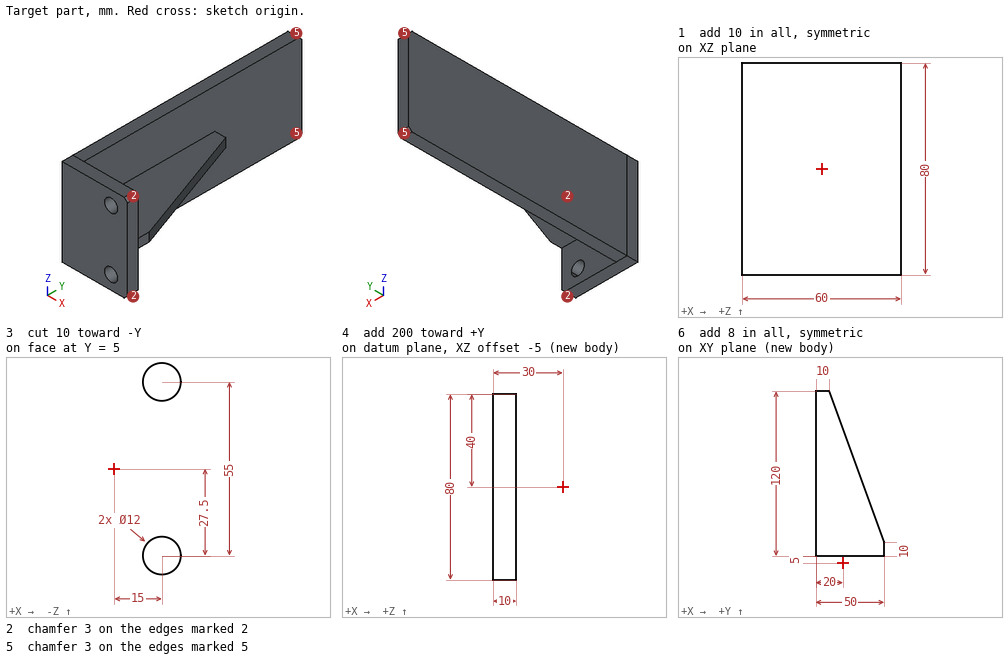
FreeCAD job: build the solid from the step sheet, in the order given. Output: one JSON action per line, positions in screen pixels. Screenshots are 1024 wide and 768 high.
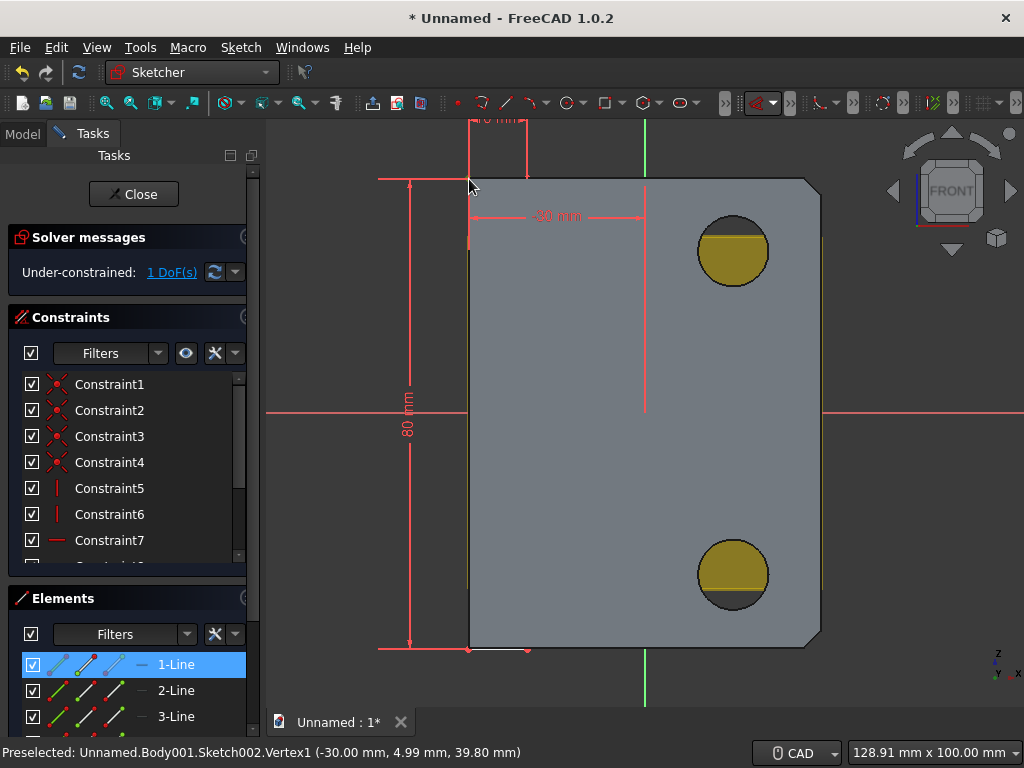
{"action": "key", "text": "i"}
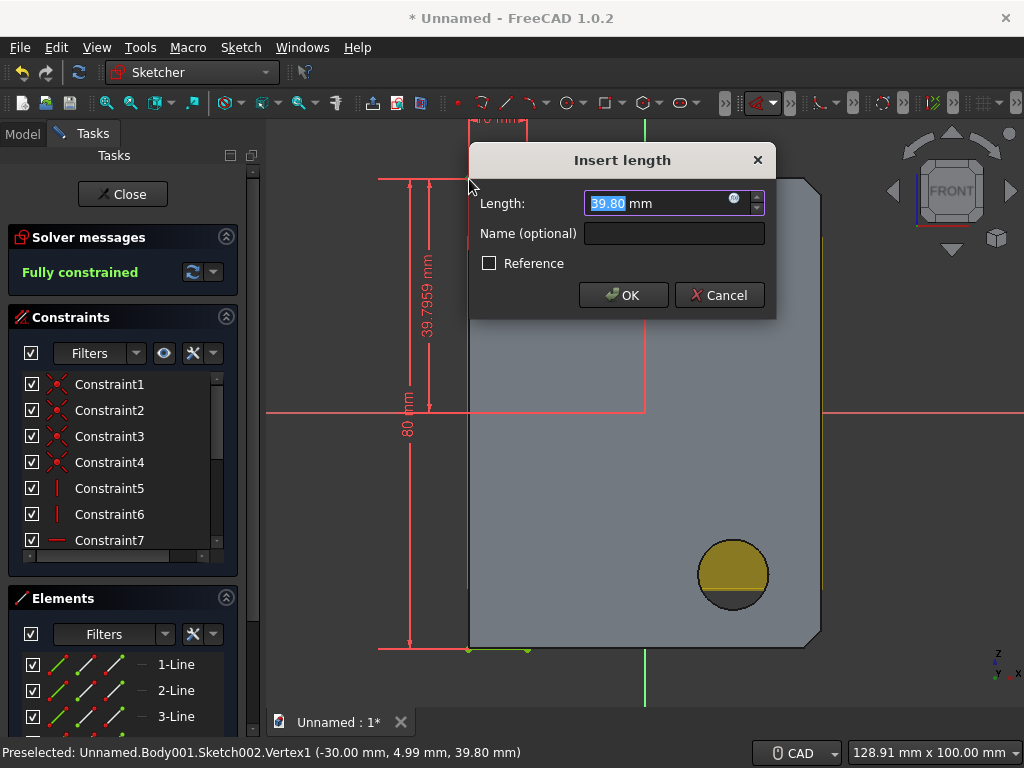
{"action": "type", "text": "40"}
{"action": "key", "text": "Return"}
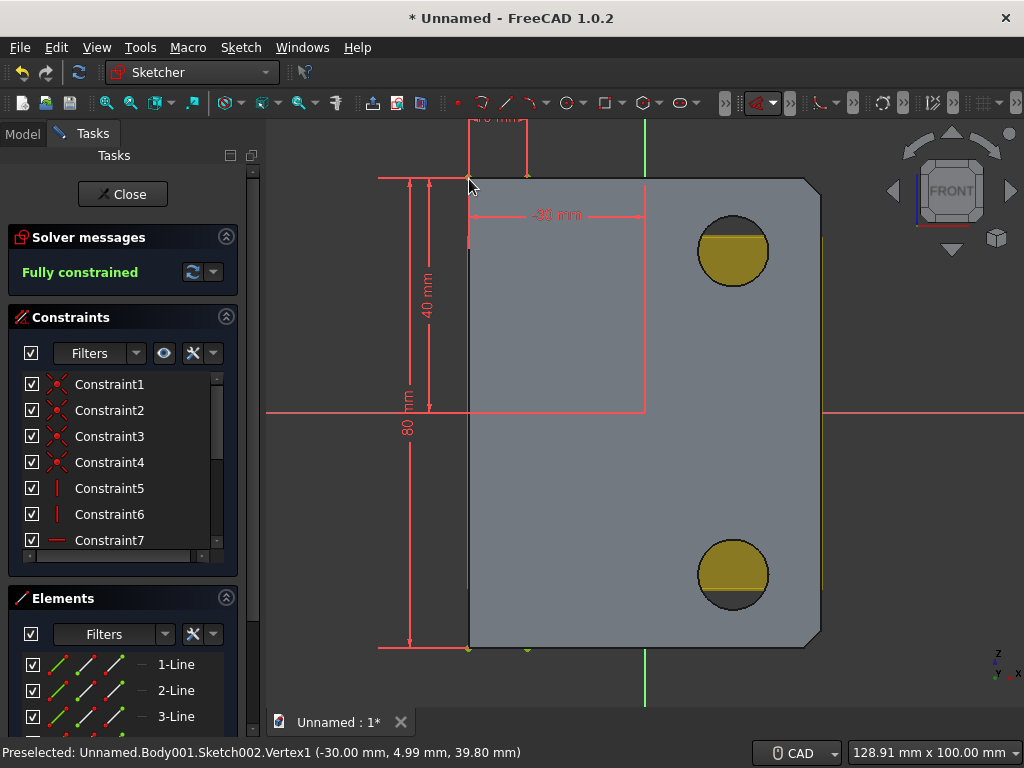
{"action": "left_click", "coordinate": [123, 194]}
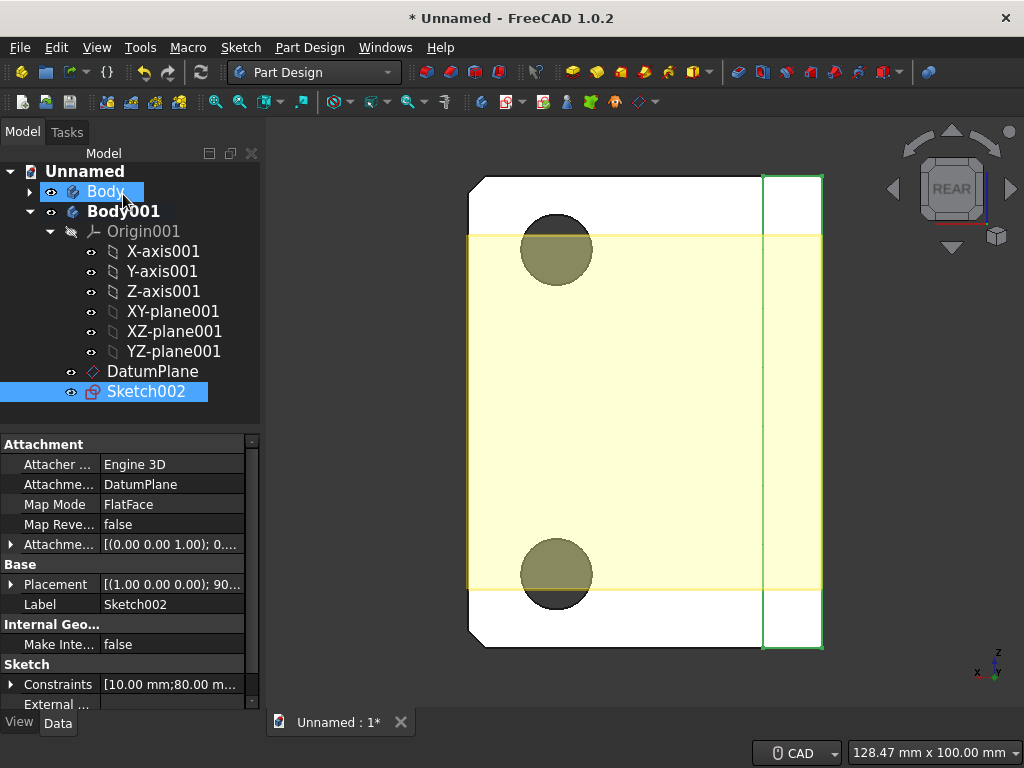
{"action": "left_click", "coordinate": [574, 72]}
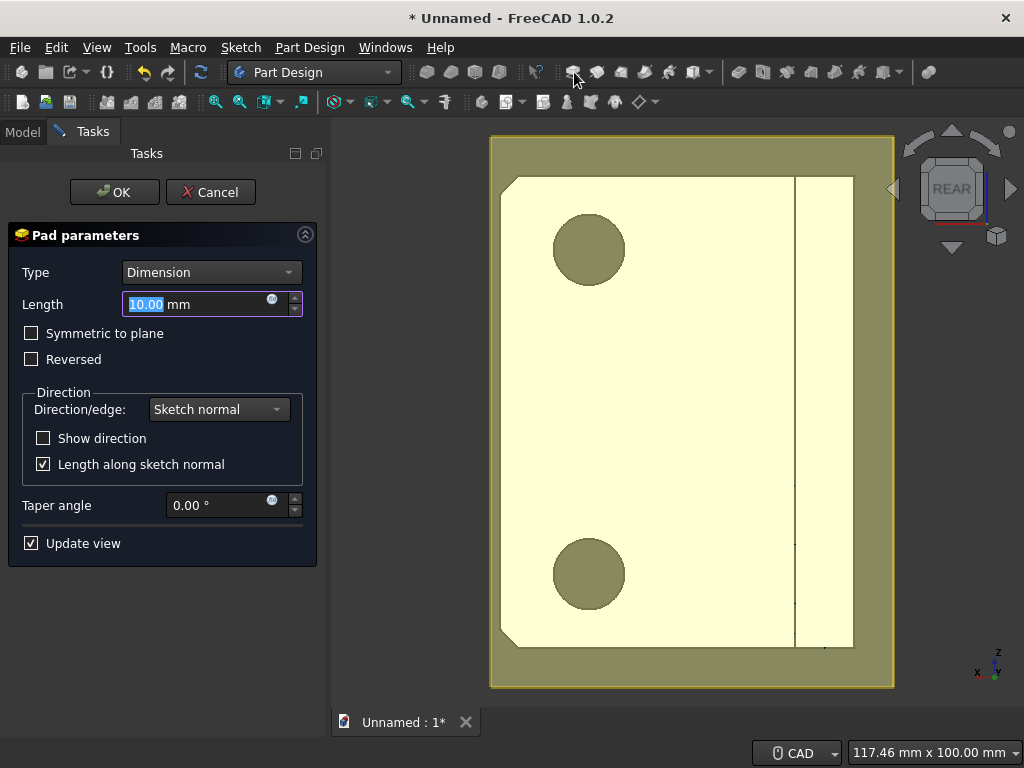
{"action": "type", "text": "200"}
{"action": "key", "text": "Tab"}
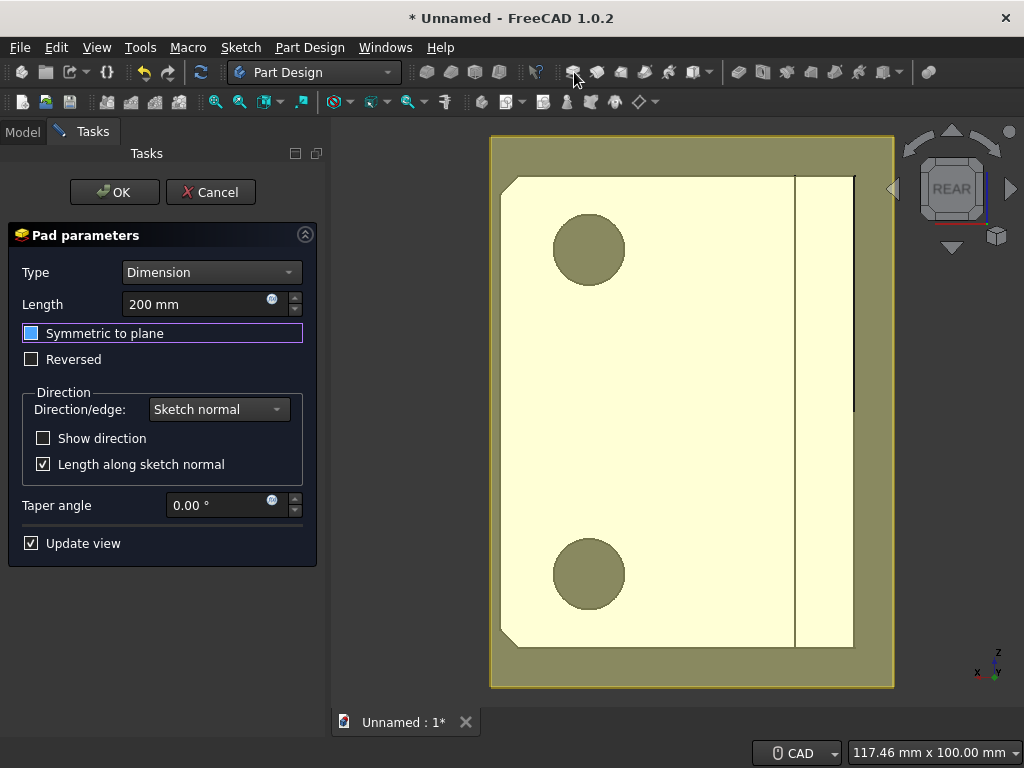
{"action": "left_click", "coordinate": [30, 359]}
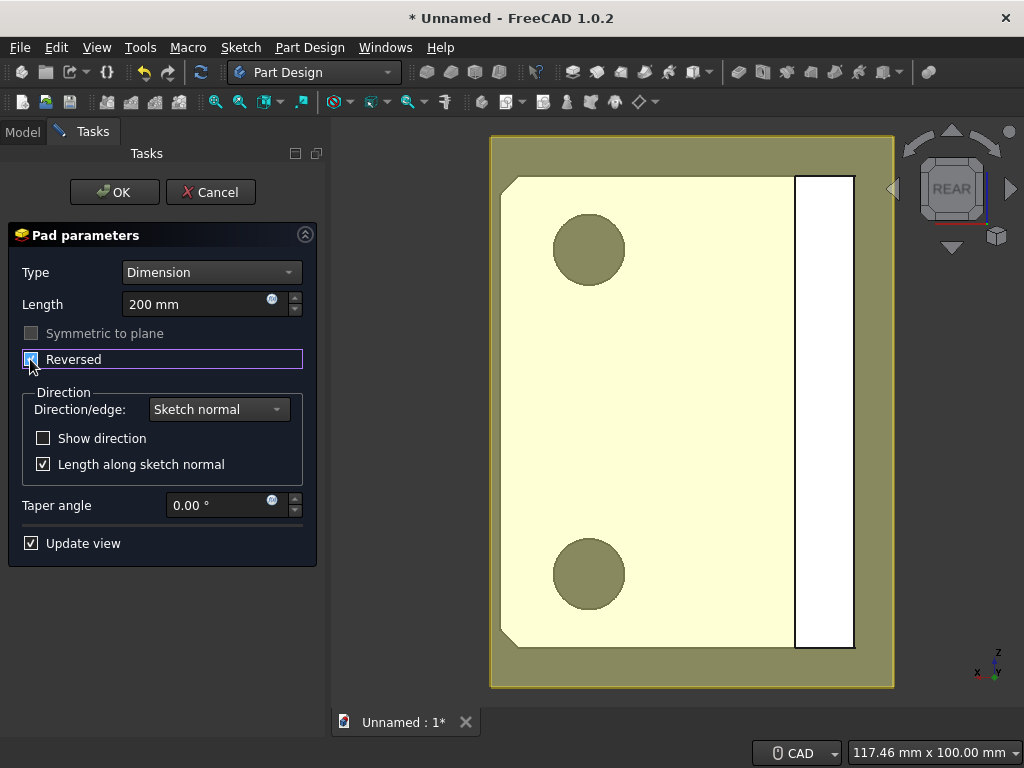
{"action": "left_click", "coordinate": [115, 192]}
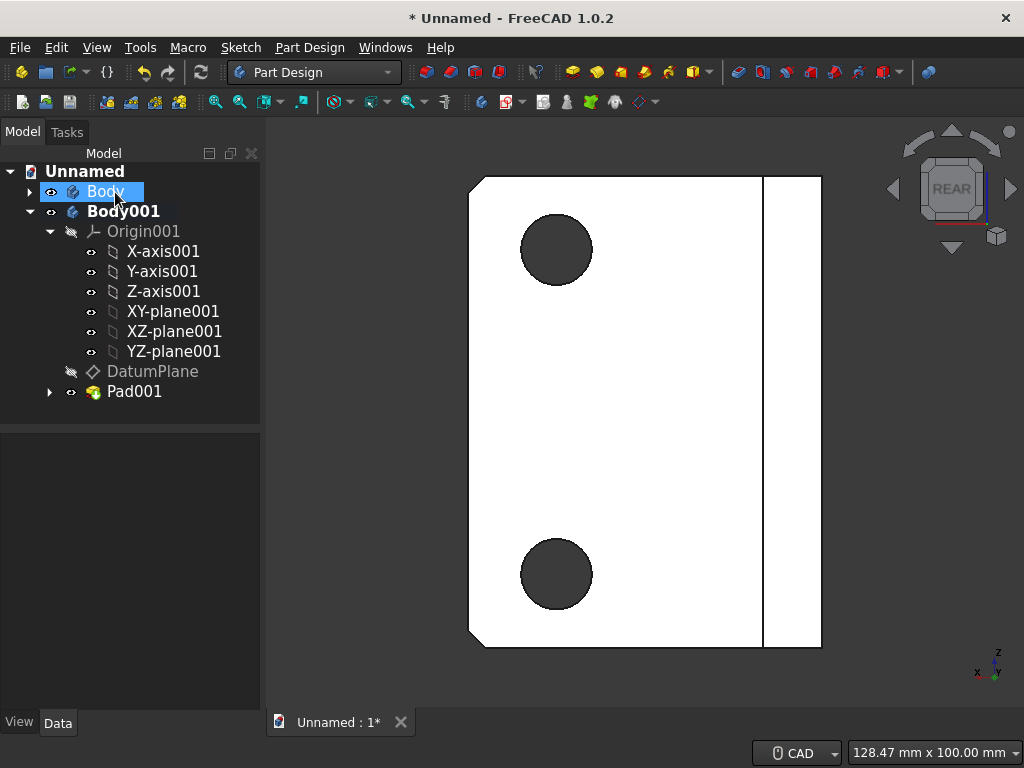
{"action": "left_click", "coordinate": [792, 647]}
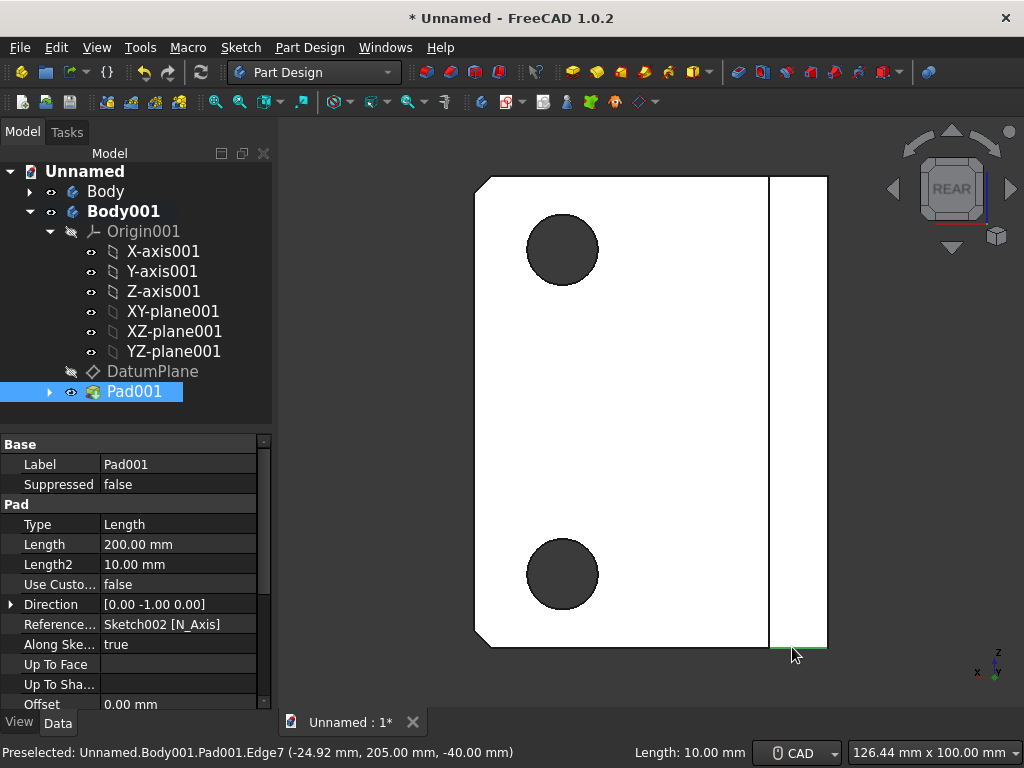
{"action": "key", "text": "0"}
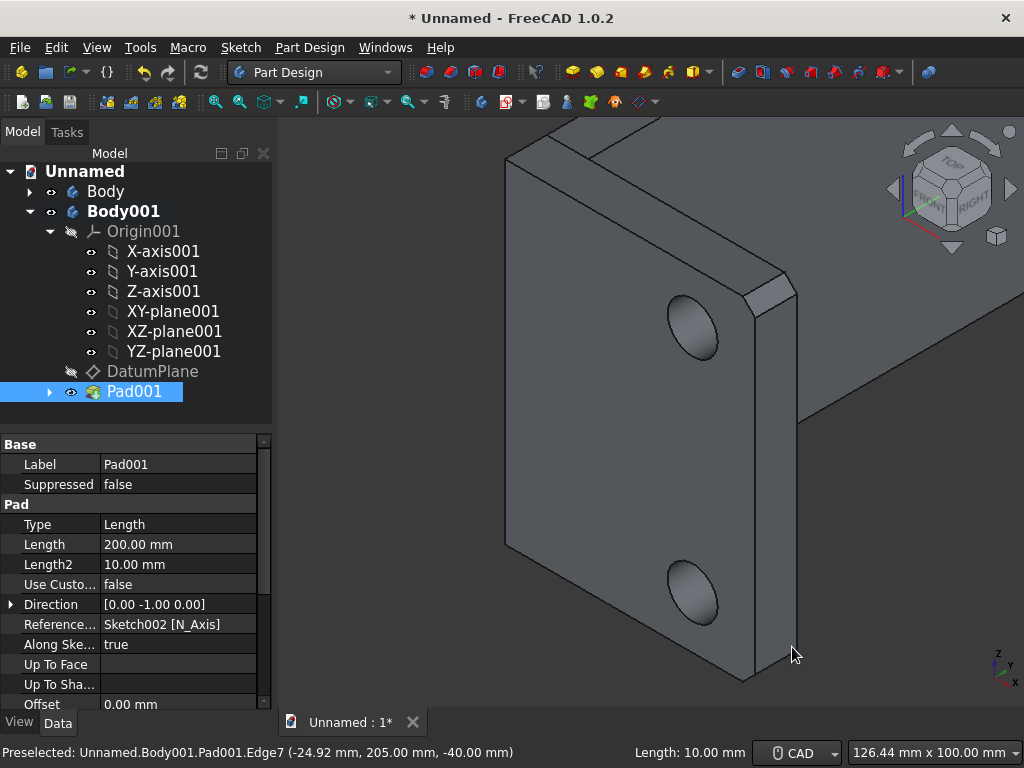
{"action": "left_click", "coordinate": [216, 102]}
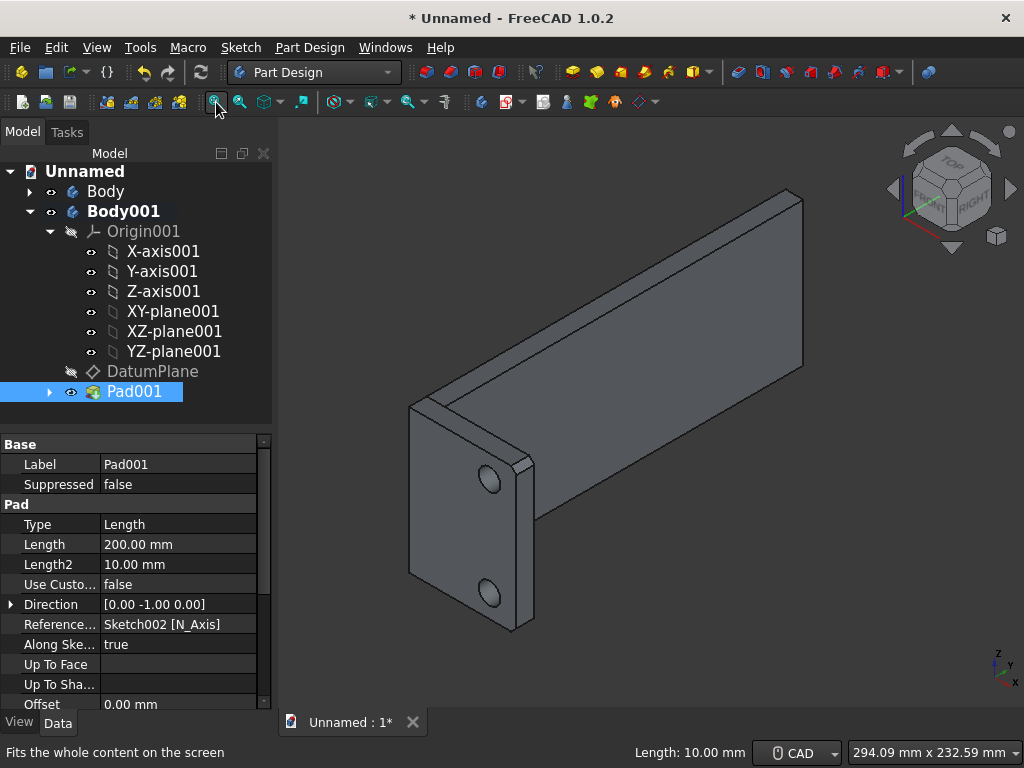
{"action": "key", "text": "2"}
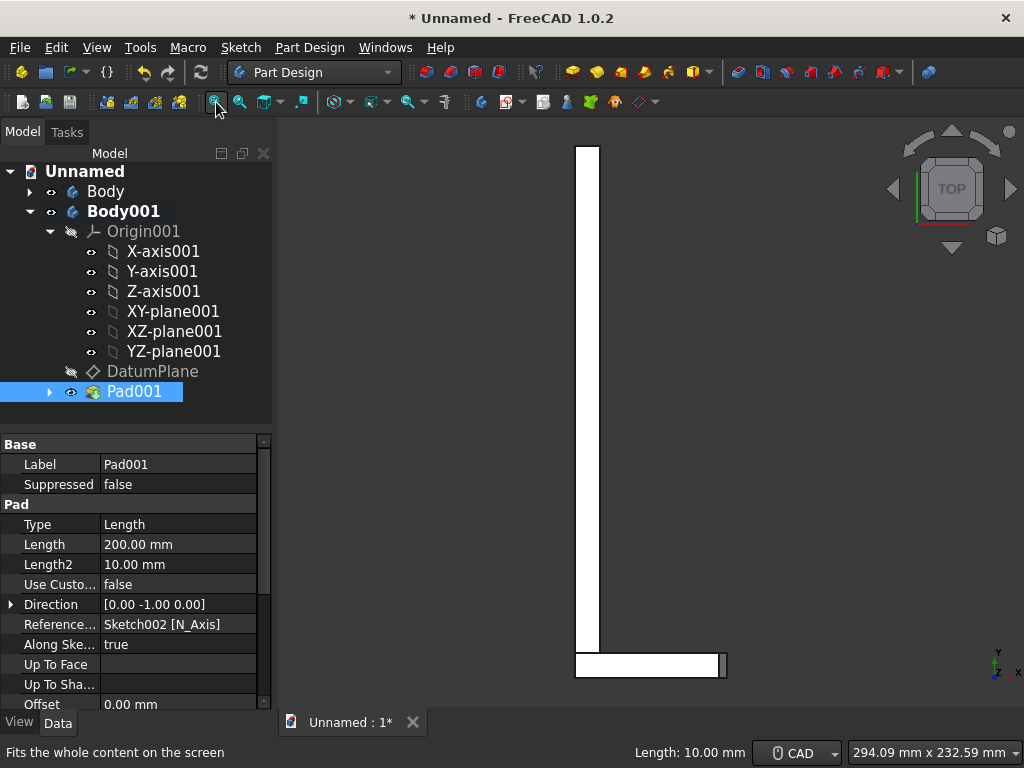
{"action": "key", "text": "1"}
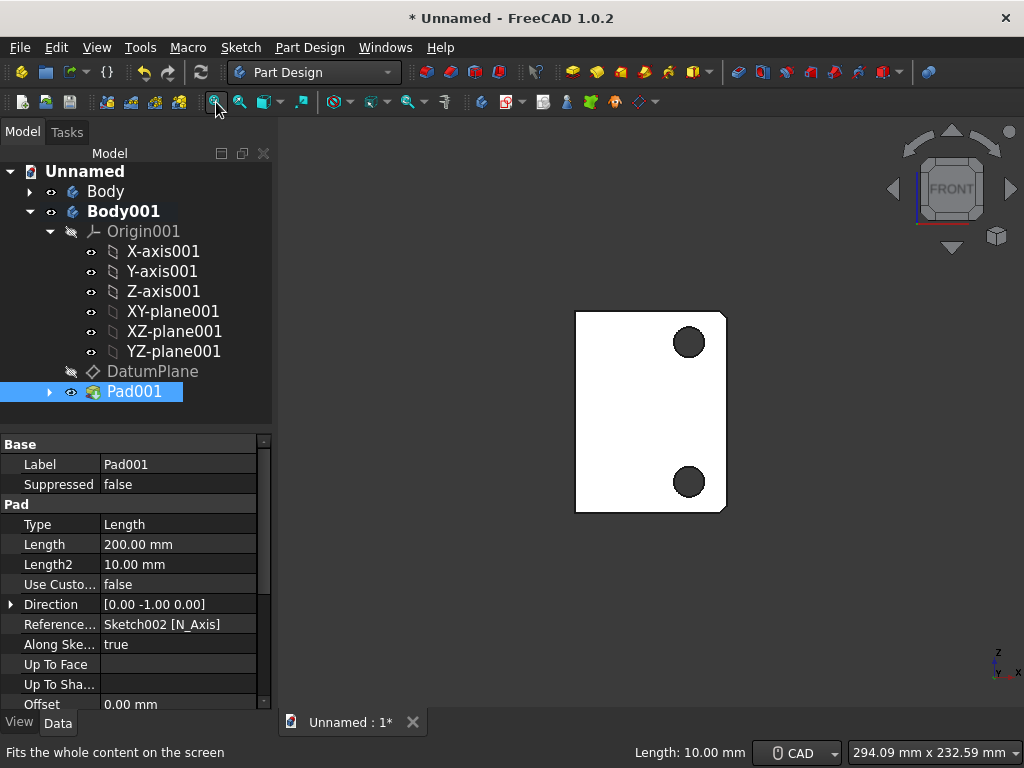
{"action": "left_click", "coordinate": [216, 102]}